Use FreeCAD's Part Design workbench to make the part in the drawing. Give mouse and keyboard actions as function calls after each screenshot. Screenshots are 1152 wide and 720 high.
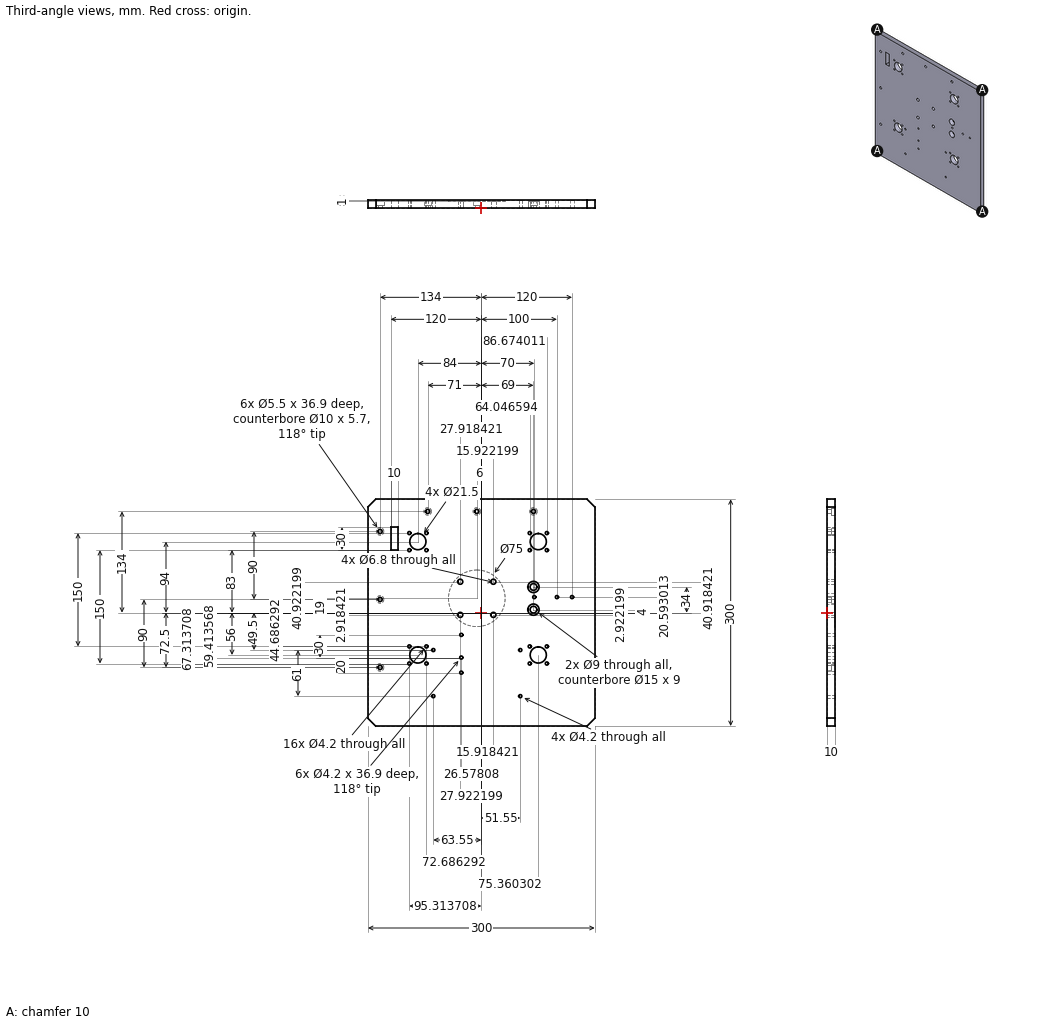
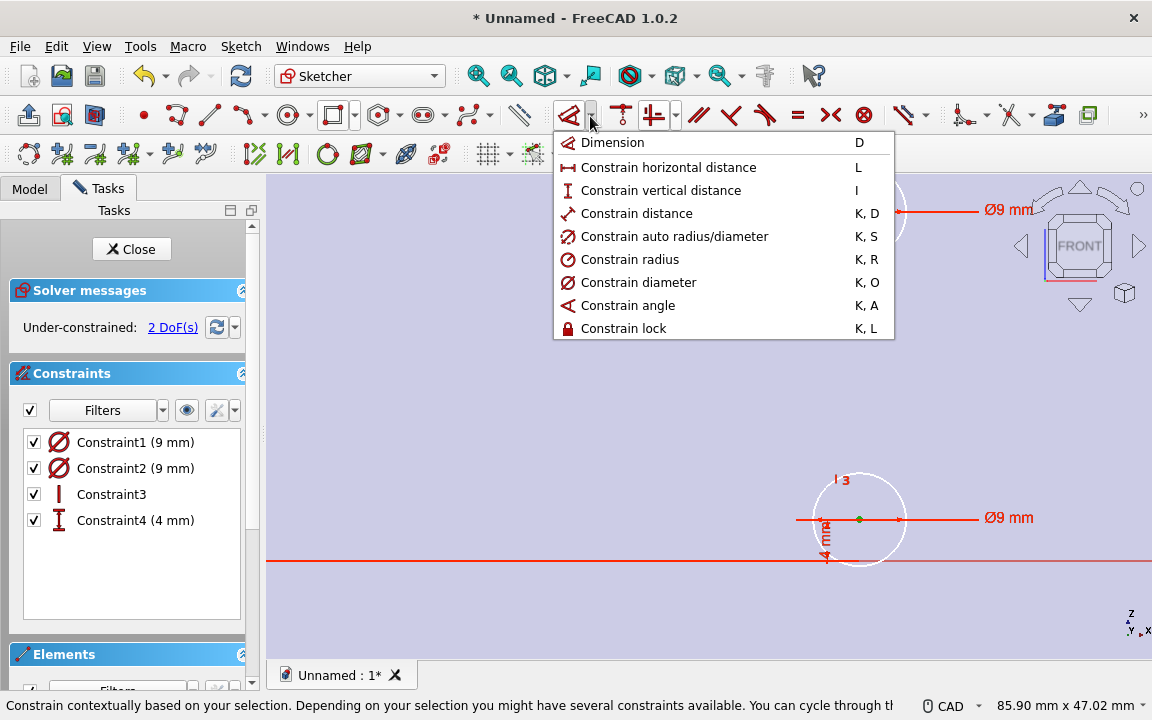
click(724, 168)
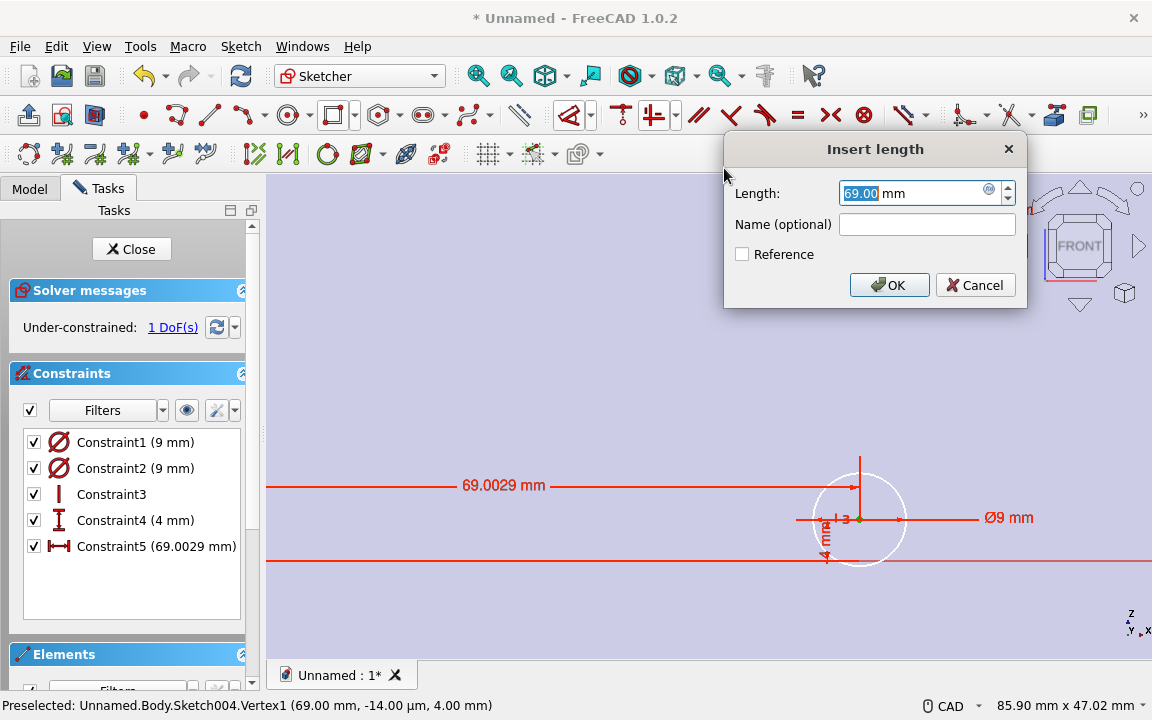
text(69)
key(Return)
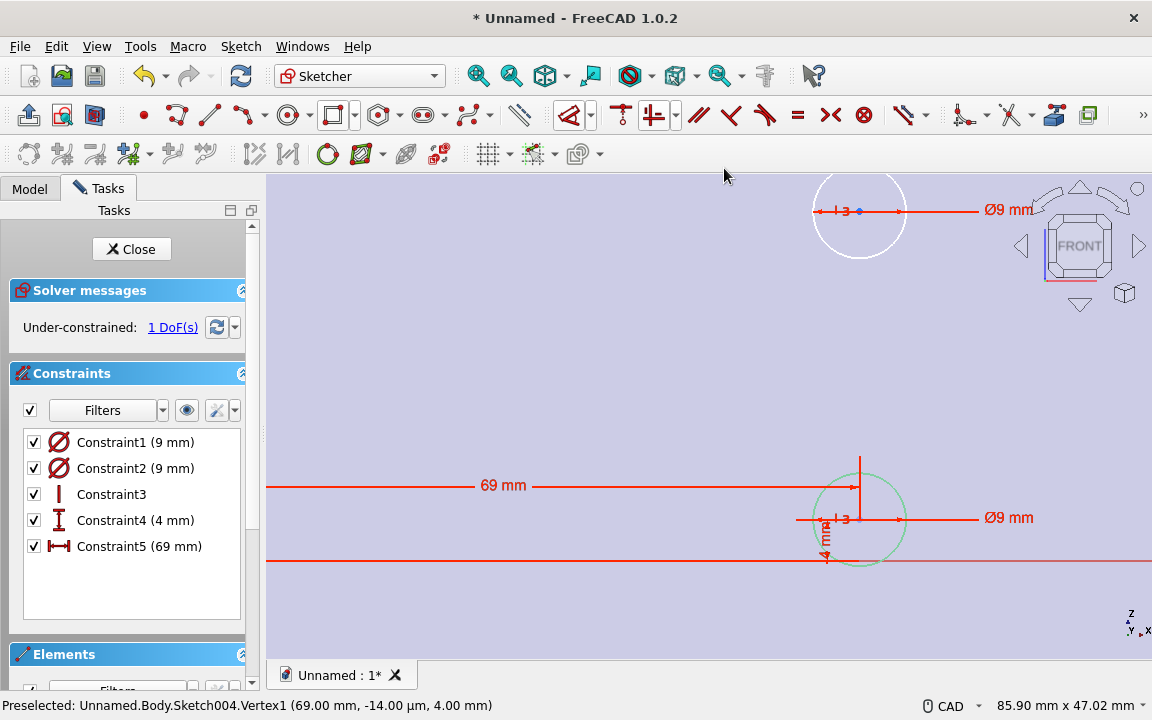
click(860, 212)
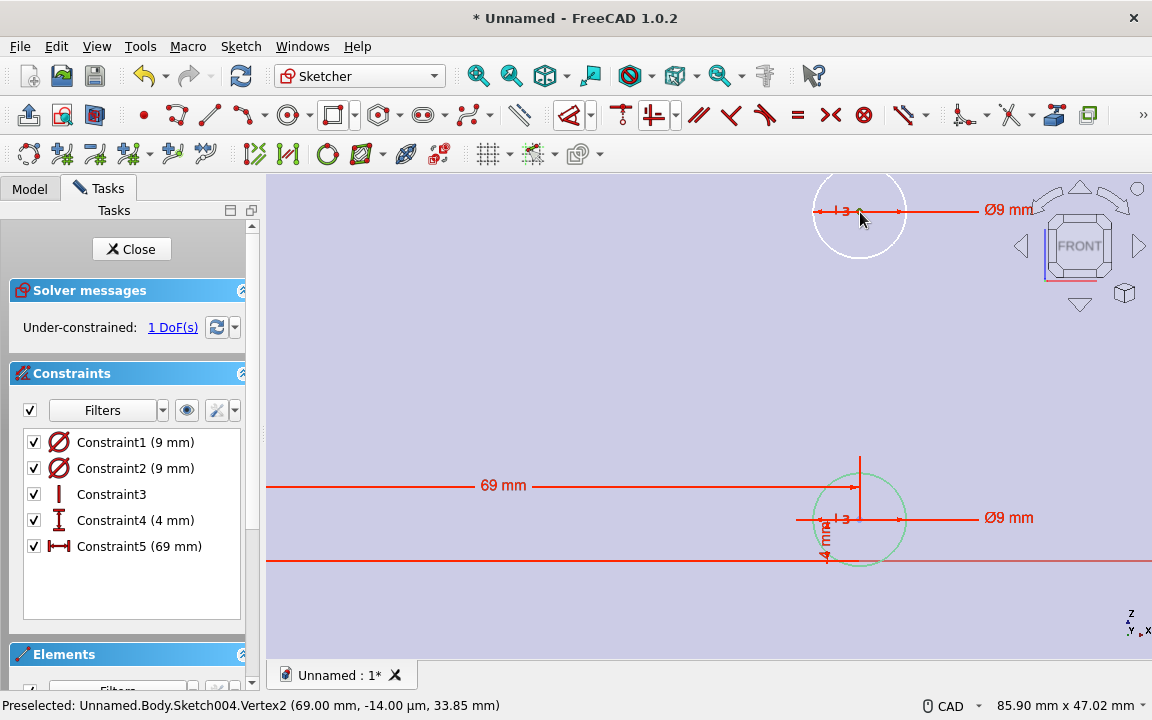
key(i)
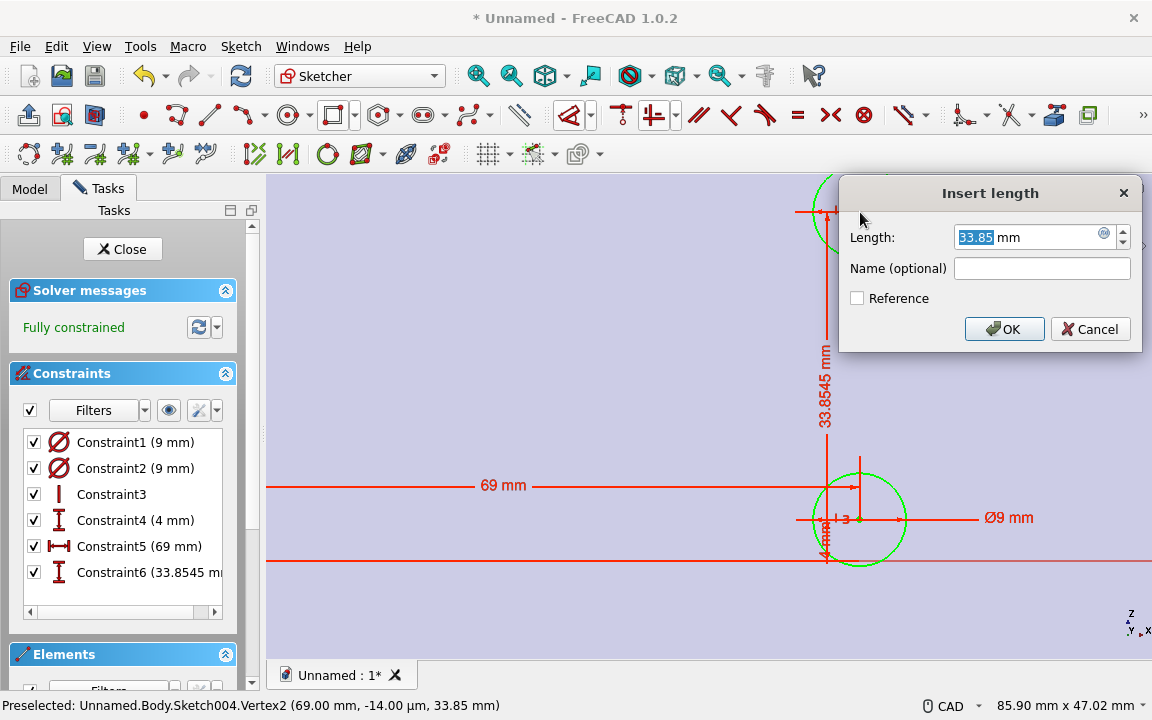
text(34)
key(Return)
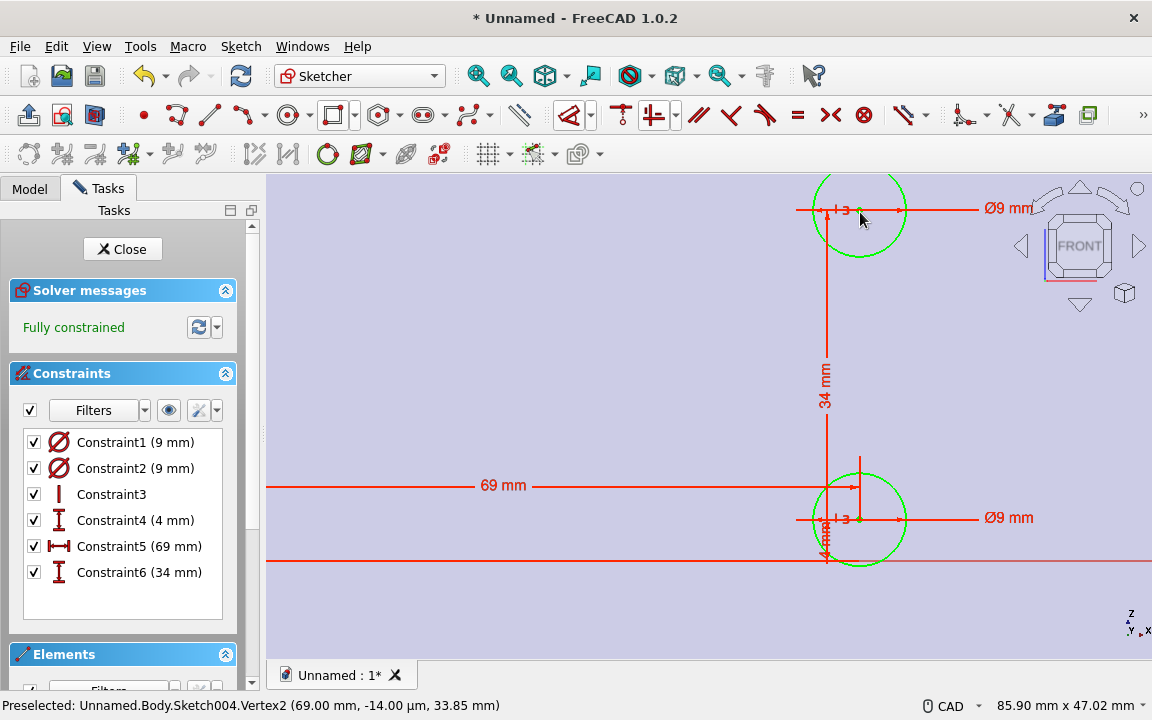
click(123, 249)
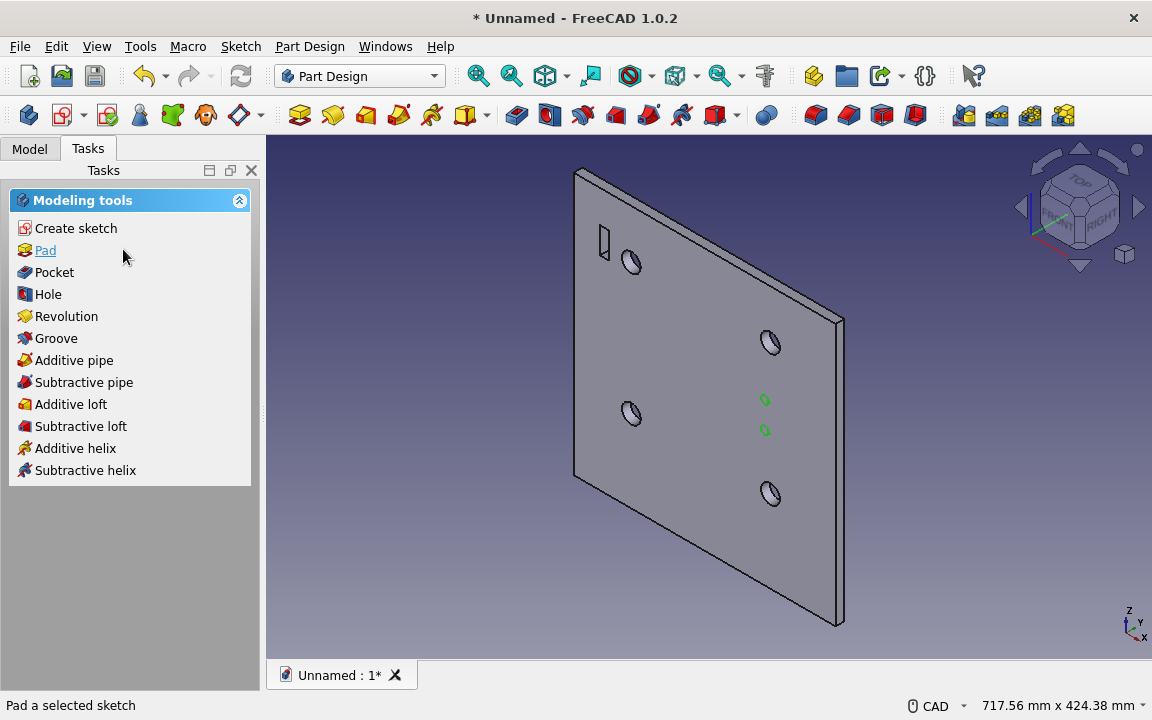
click(550, 116)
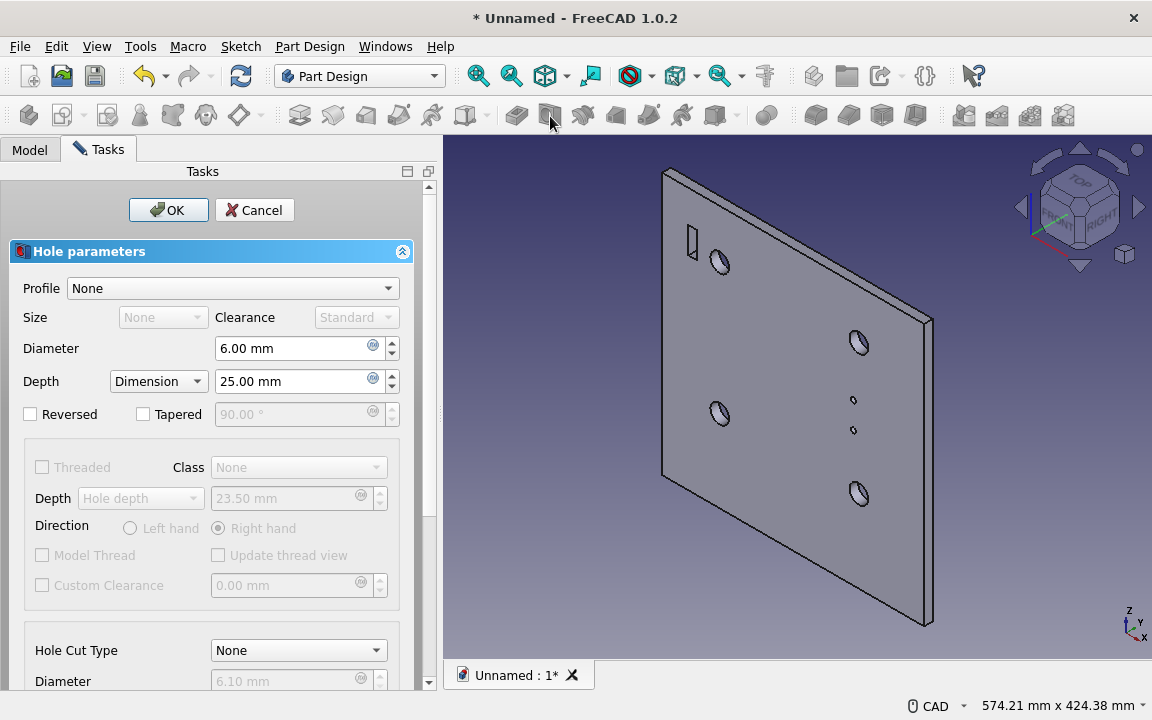
triple_click(300, 348)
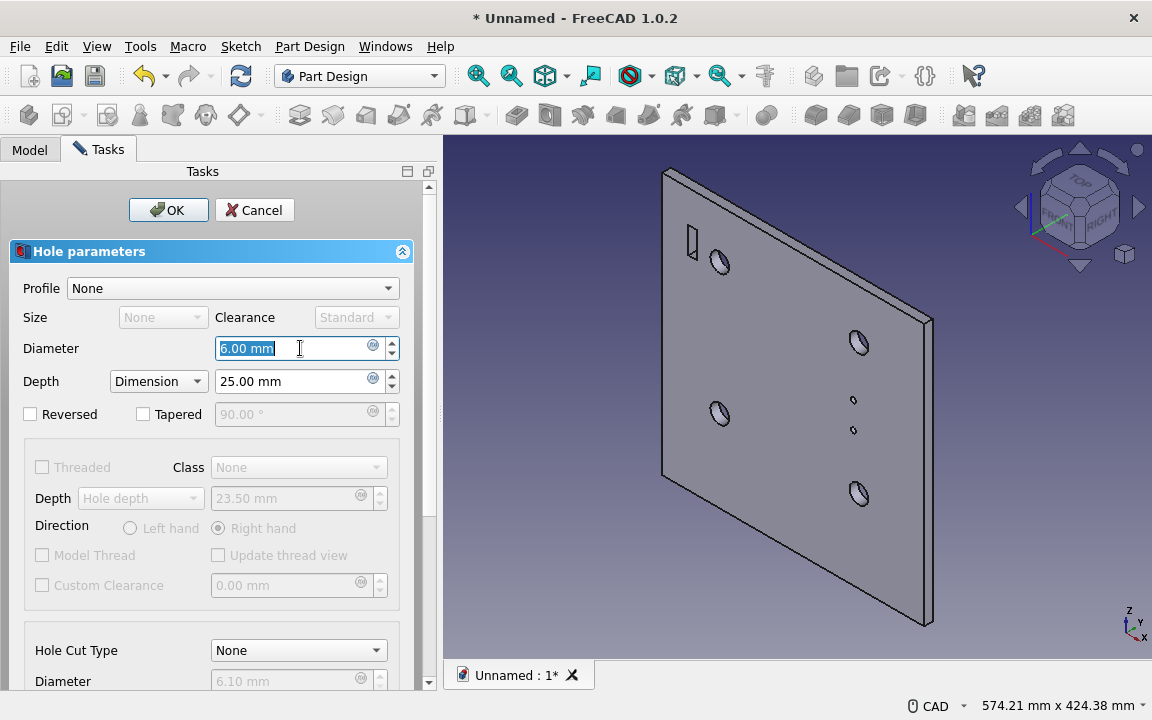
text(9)
key(Tab)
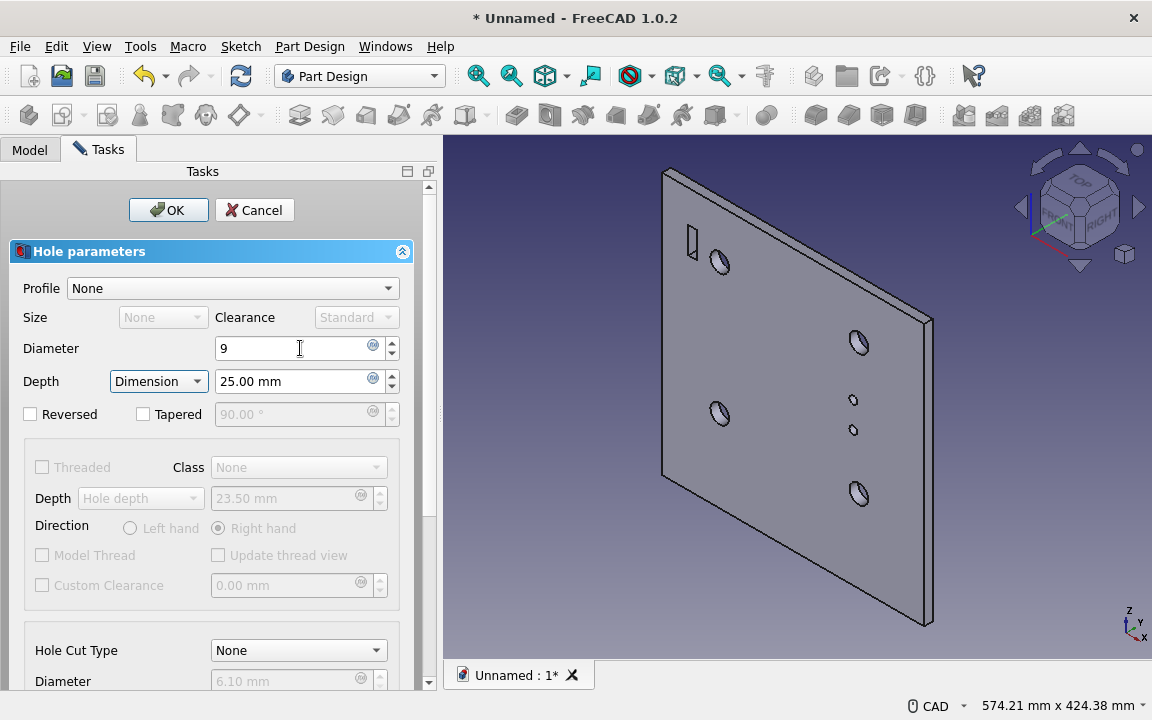
click(160, 382)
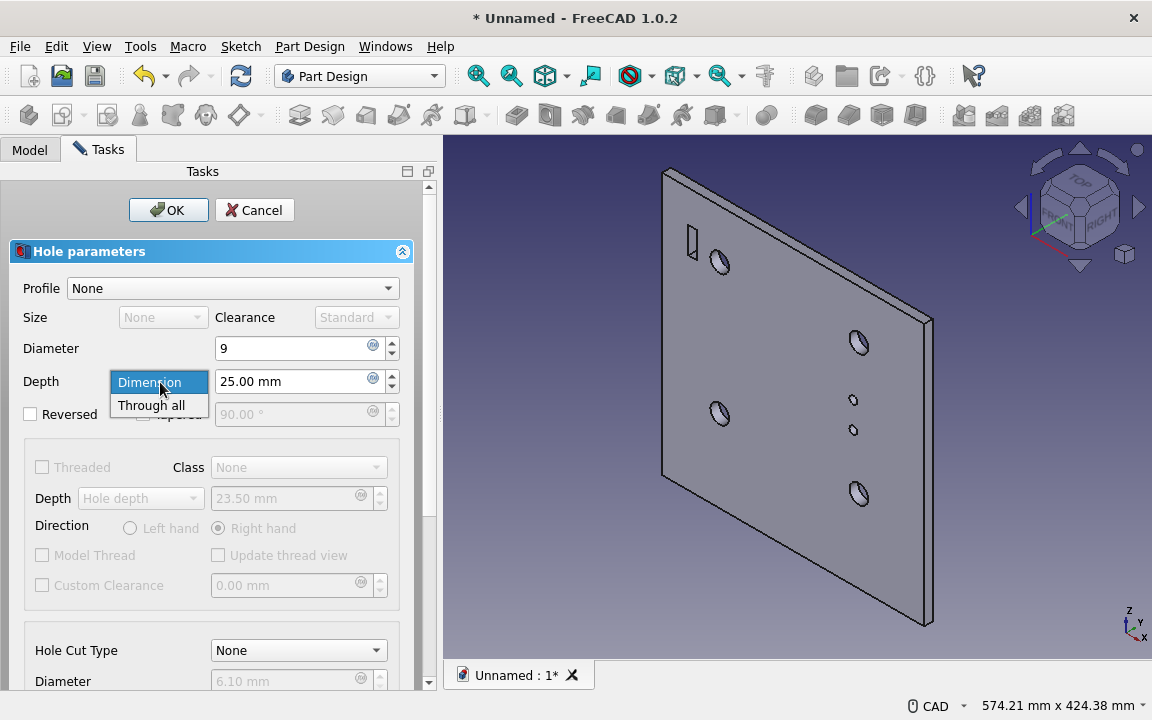
click(158, 406)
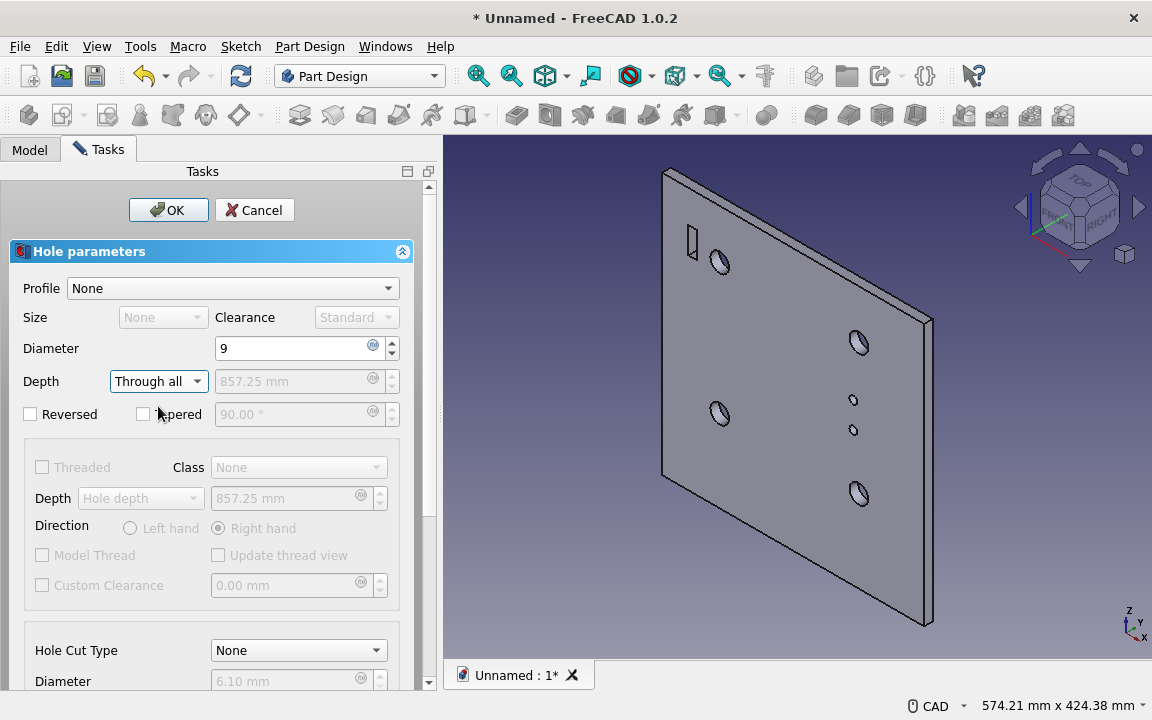
click(300, 650)